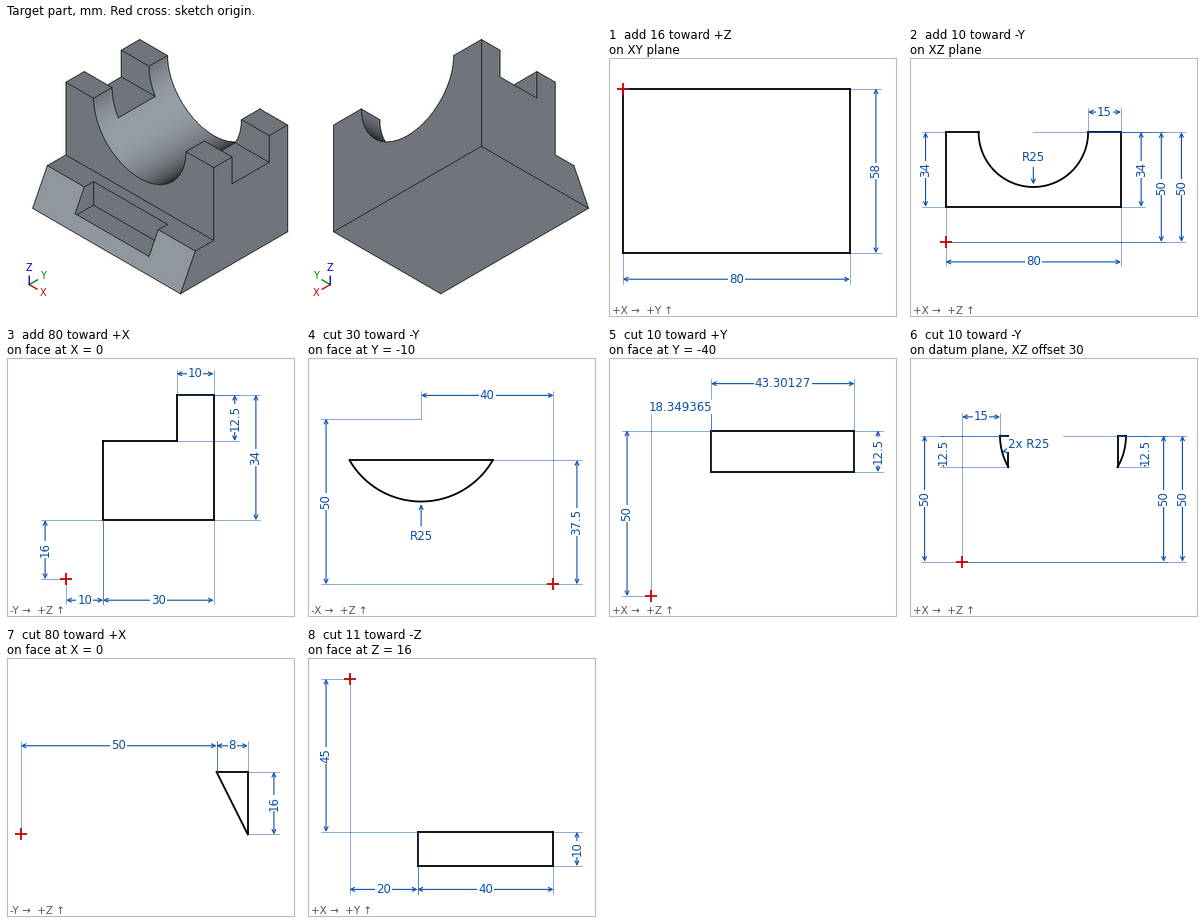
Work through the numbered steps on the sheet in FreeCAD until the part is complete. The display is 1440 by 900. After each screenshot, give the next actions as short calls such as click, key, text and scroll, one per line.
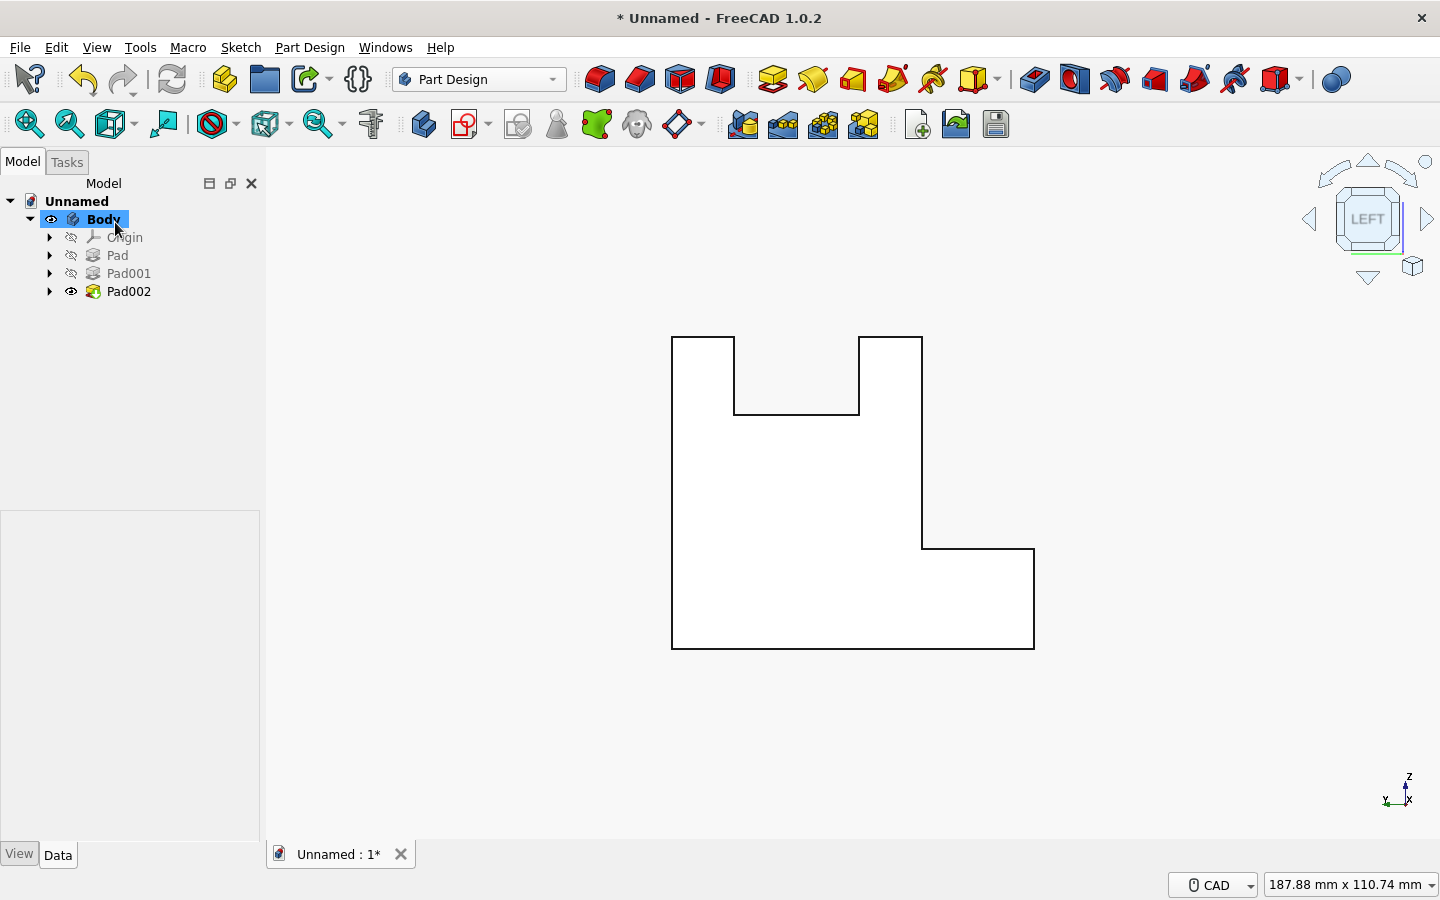
key(4)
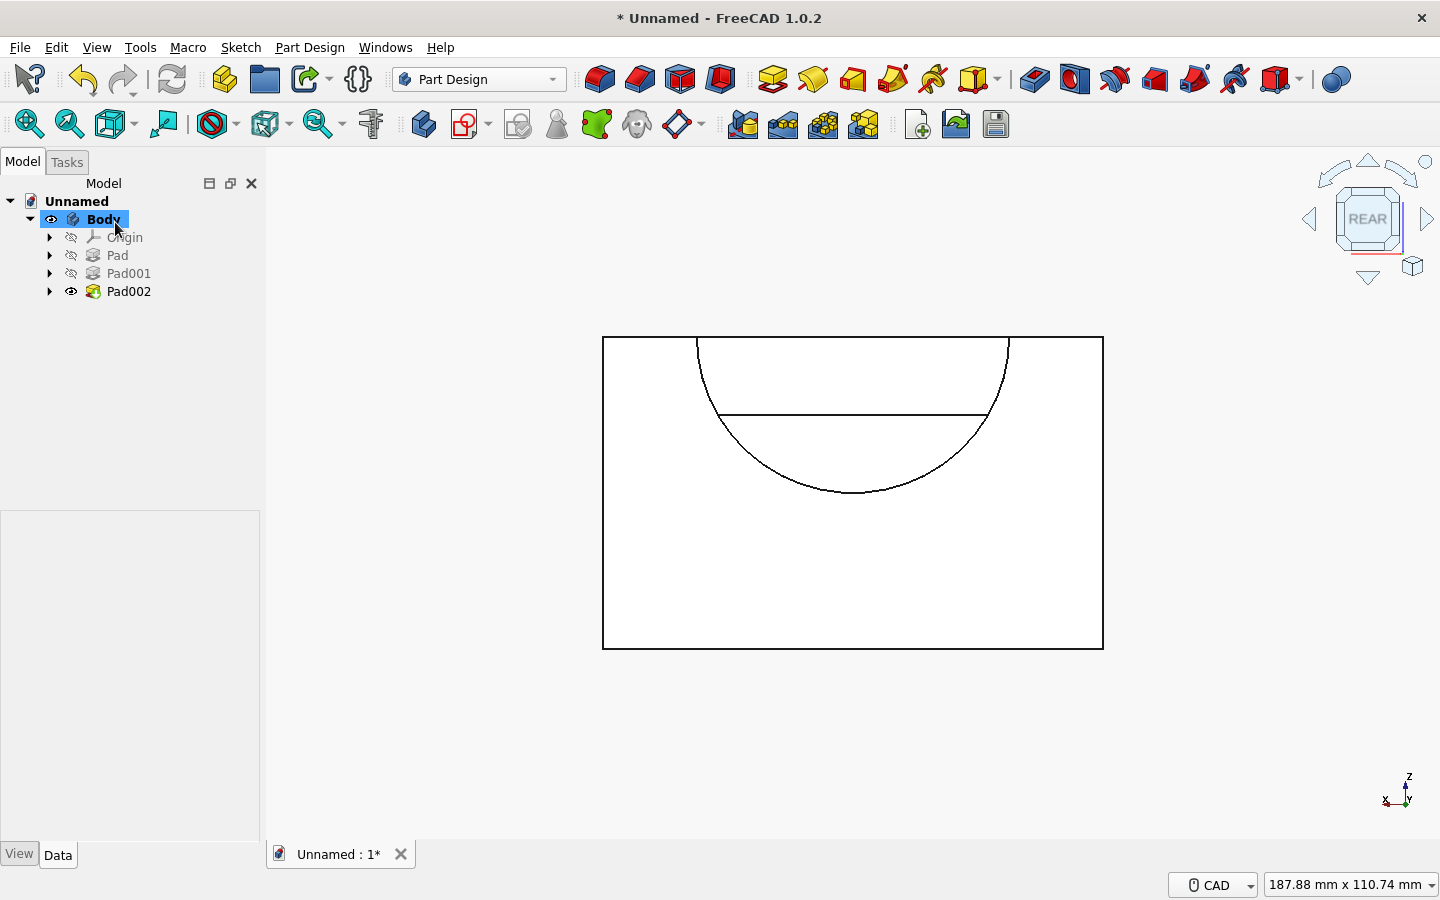
click(853, 453)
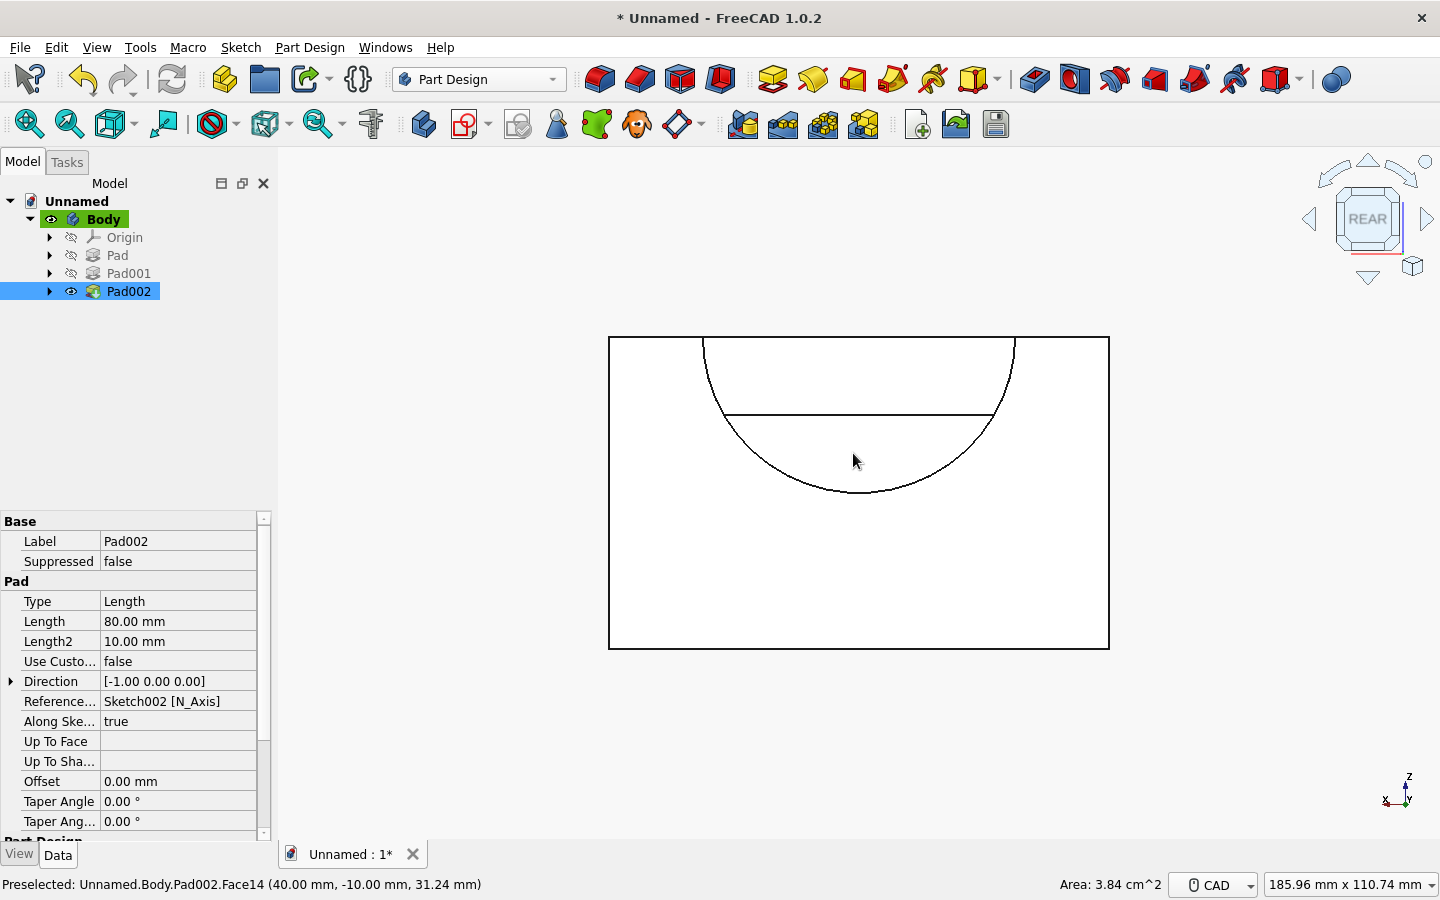
click(464, 124)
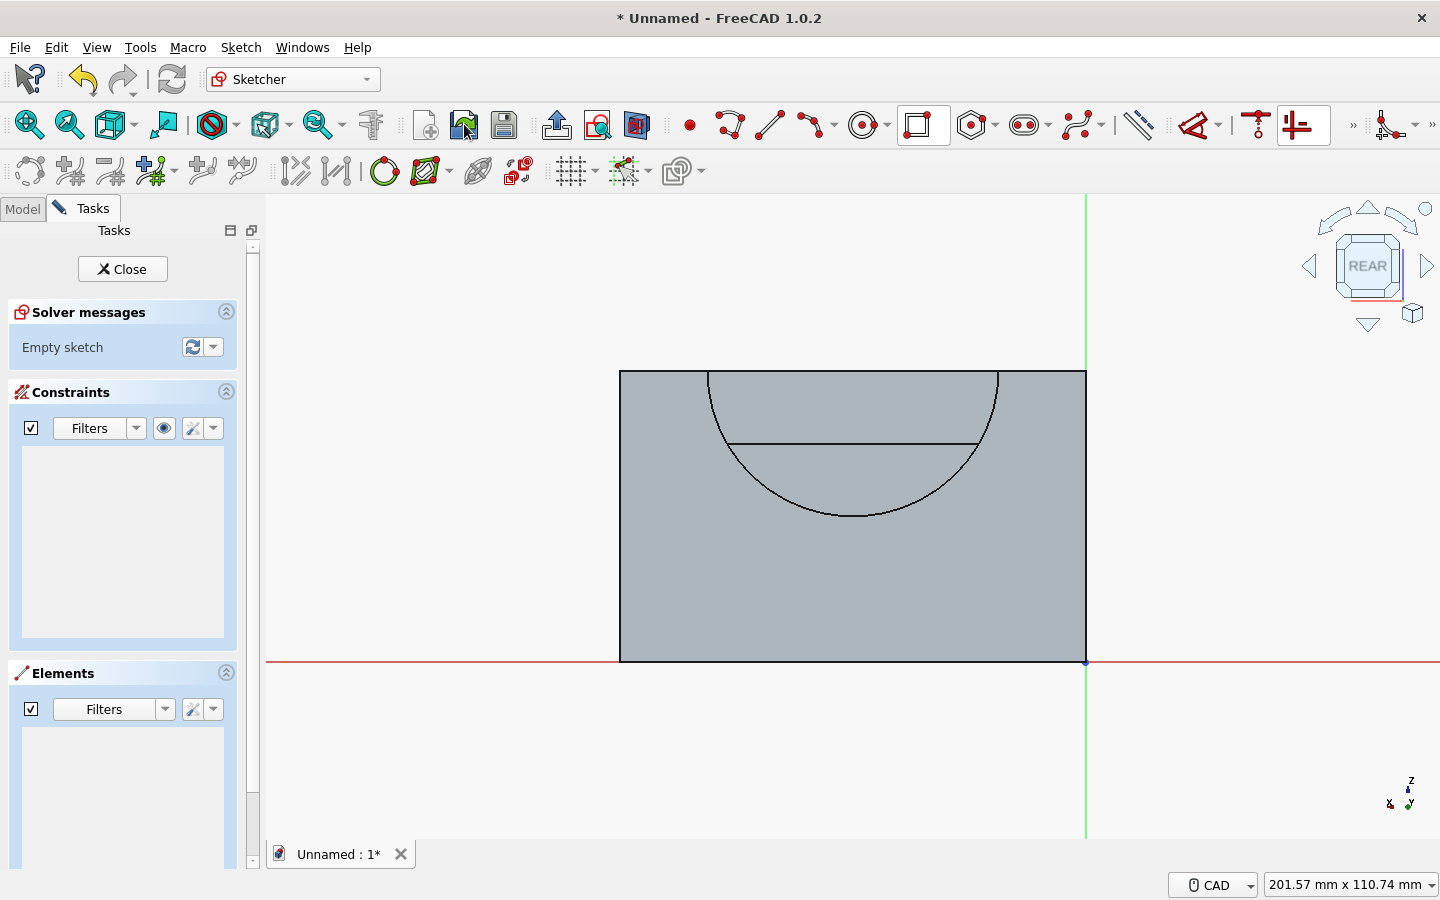
scroll(1055, 597, up, 3)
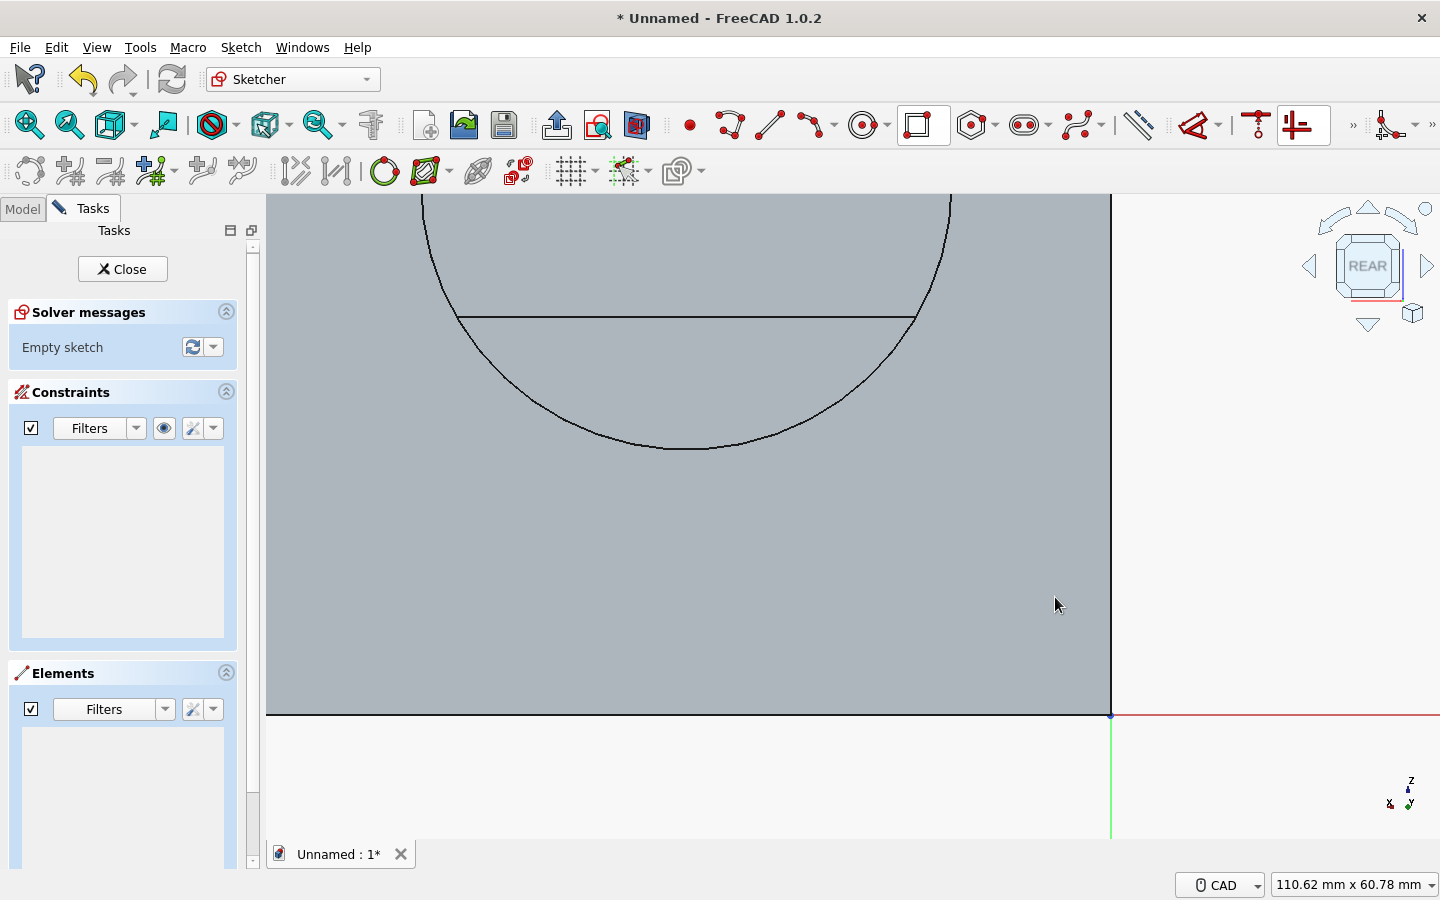
click(770, 126)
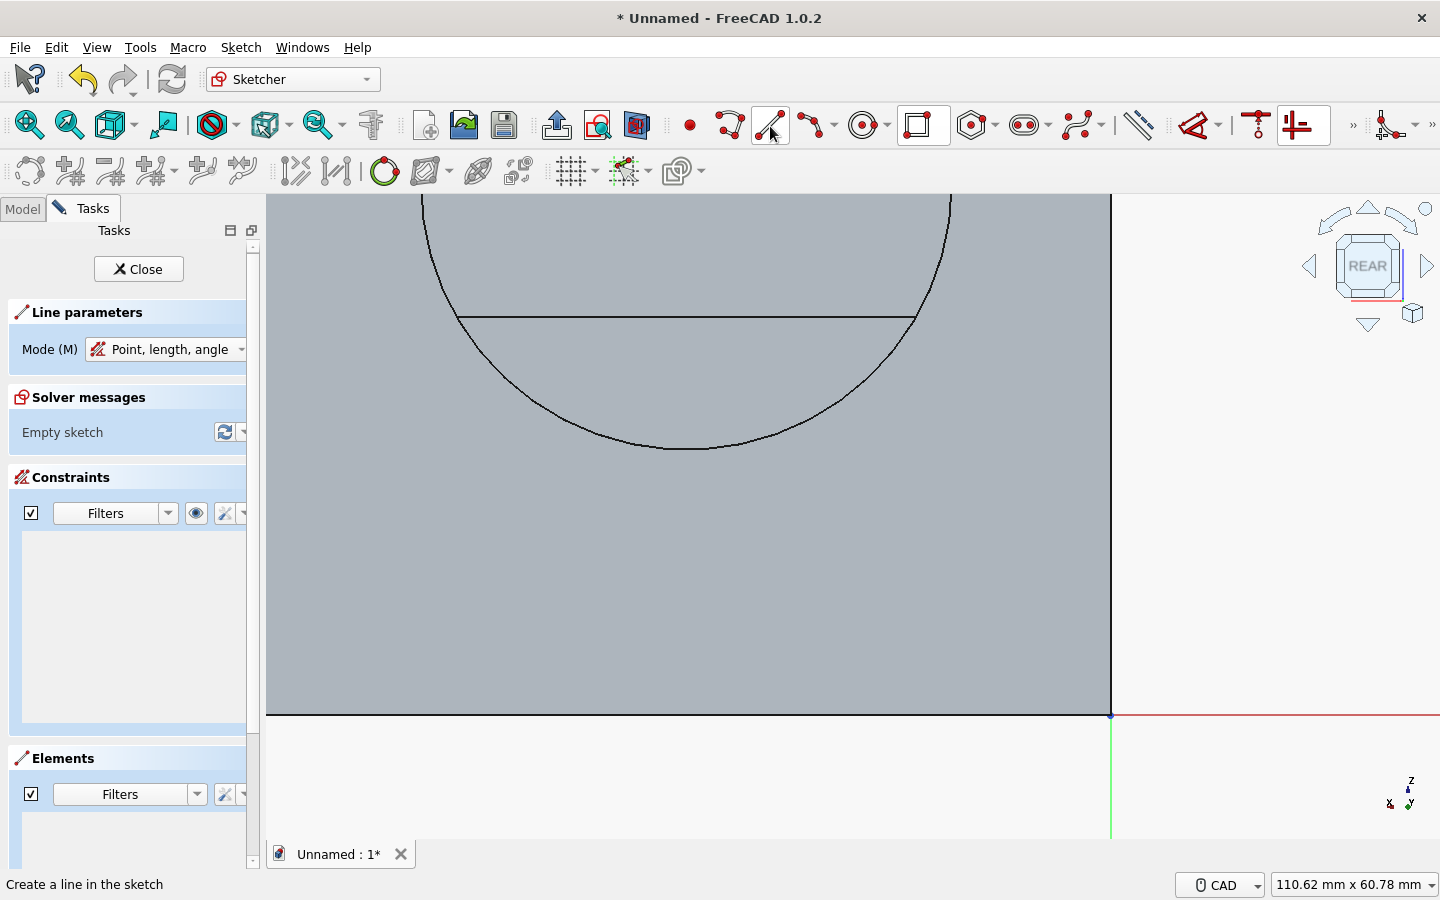
click(916, 317)
click(457, 317)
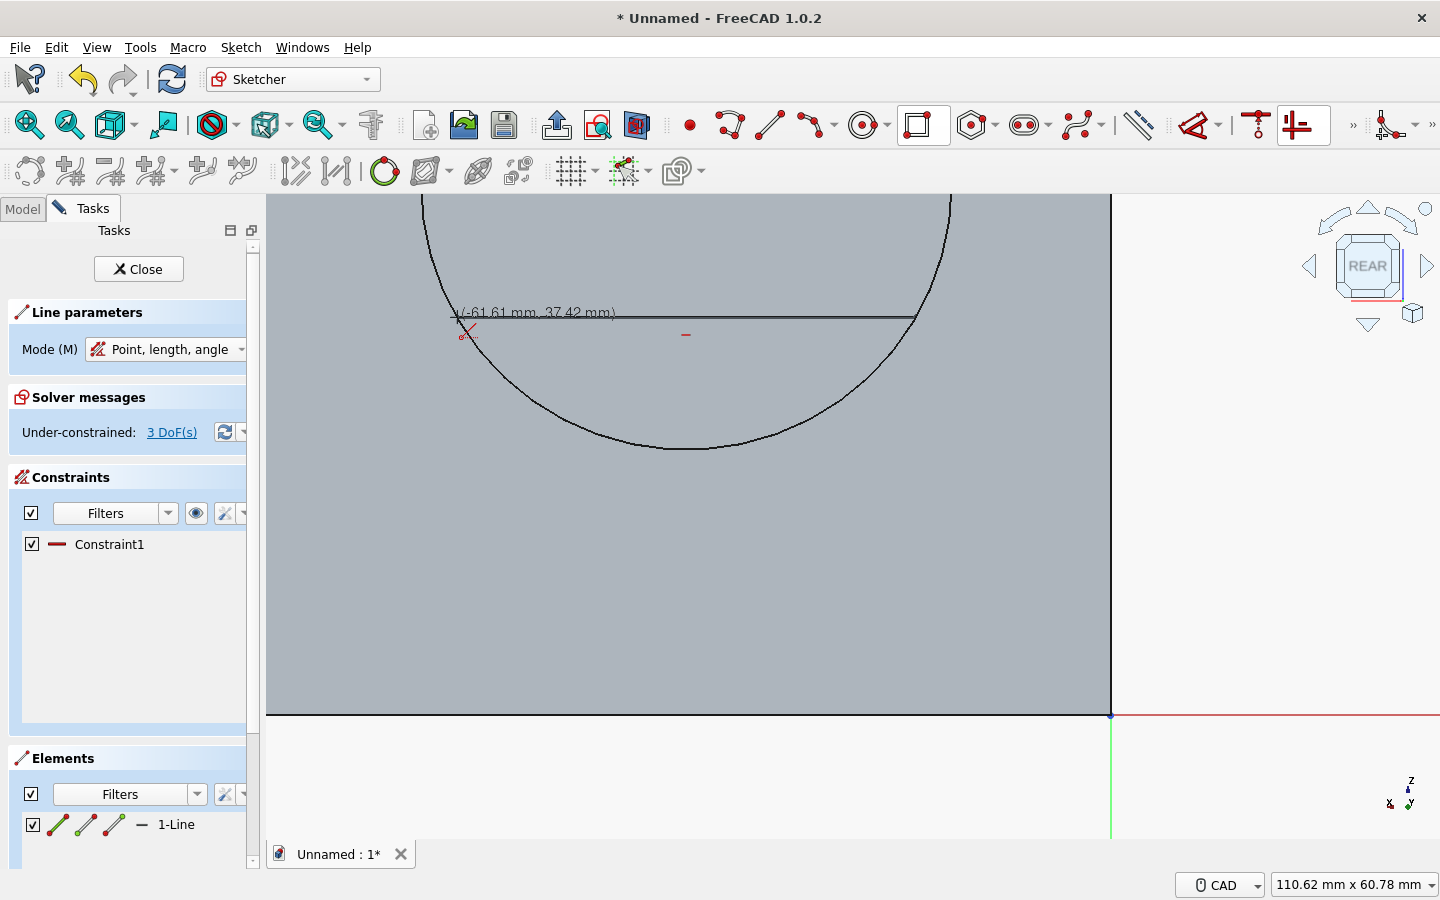
click(810, 126)